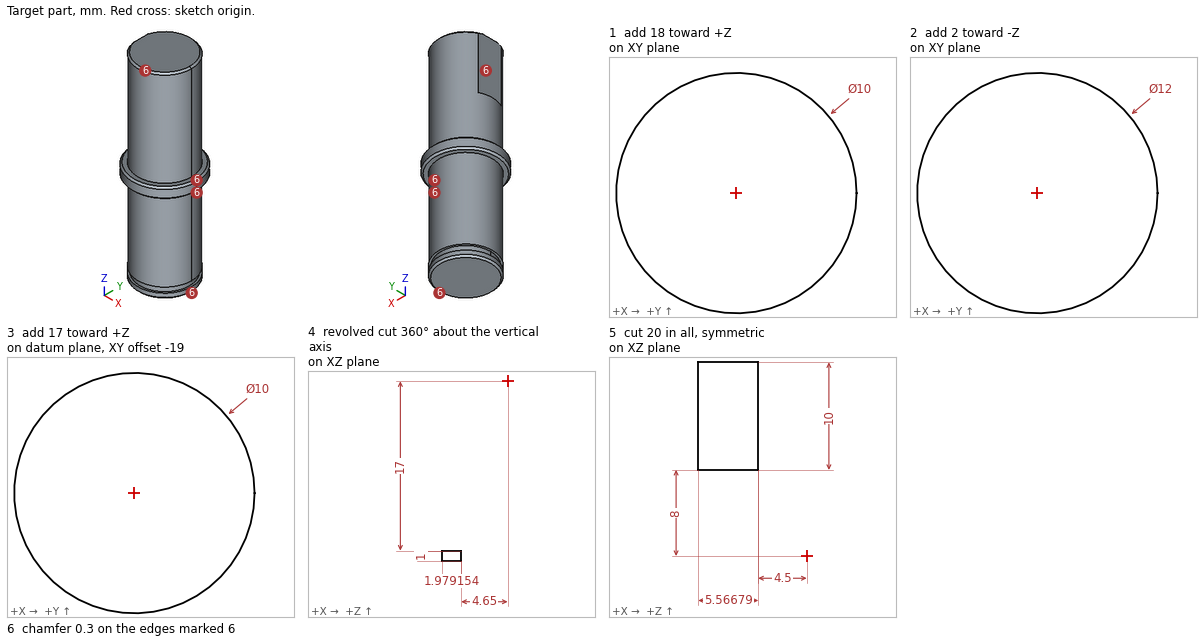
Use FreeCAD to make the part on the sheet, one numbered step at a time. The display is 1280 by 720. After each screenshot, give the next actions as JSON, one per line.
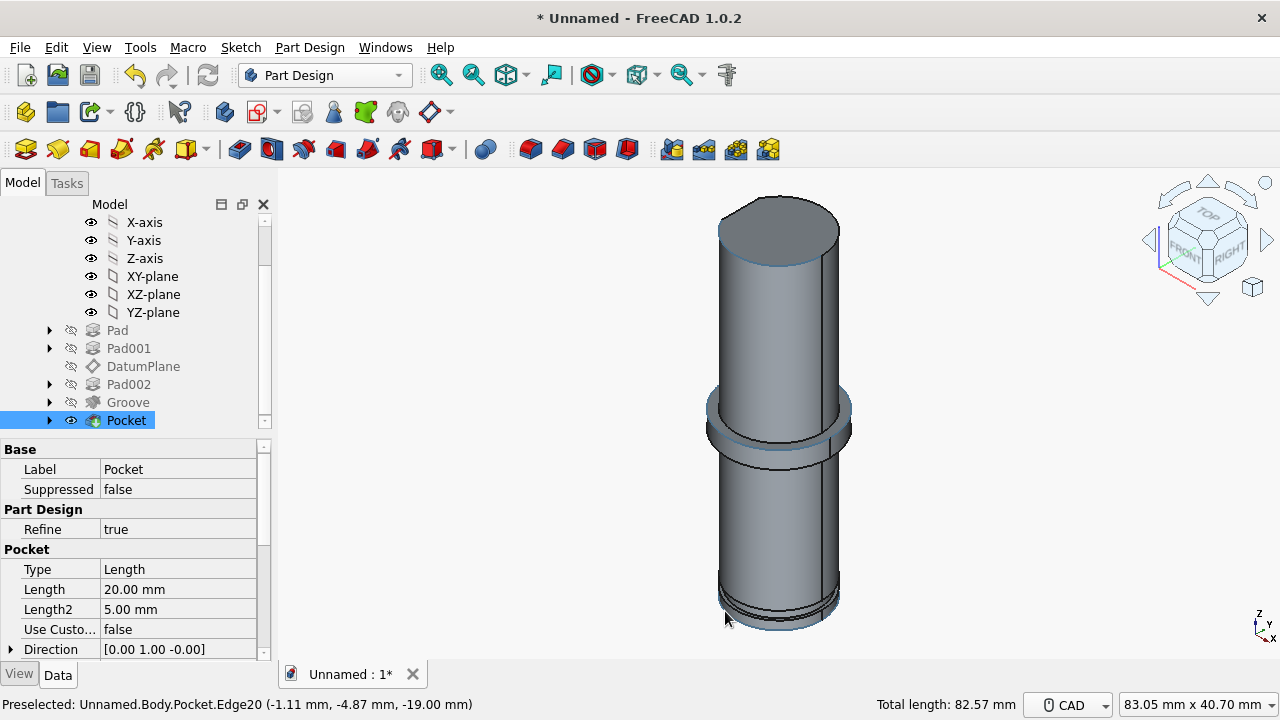
{"action": "key", "text": "2"}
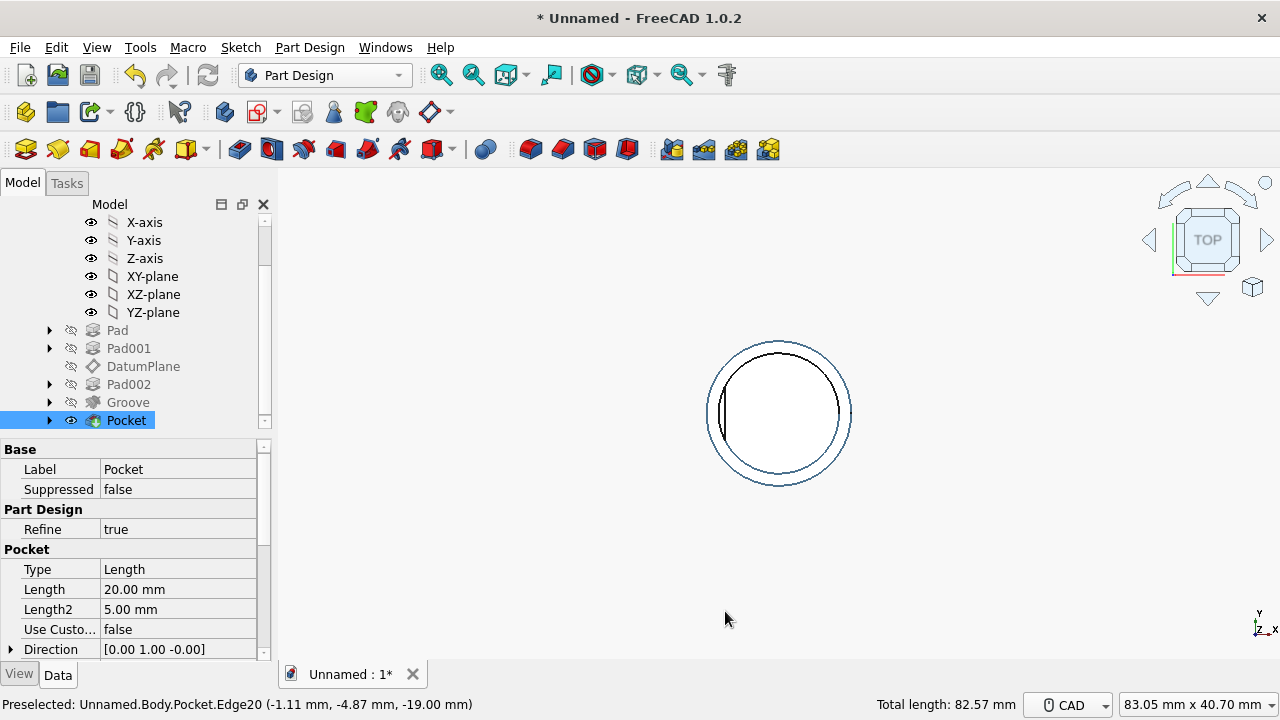
{"action": "left_click", "coordinate": [442, 76]}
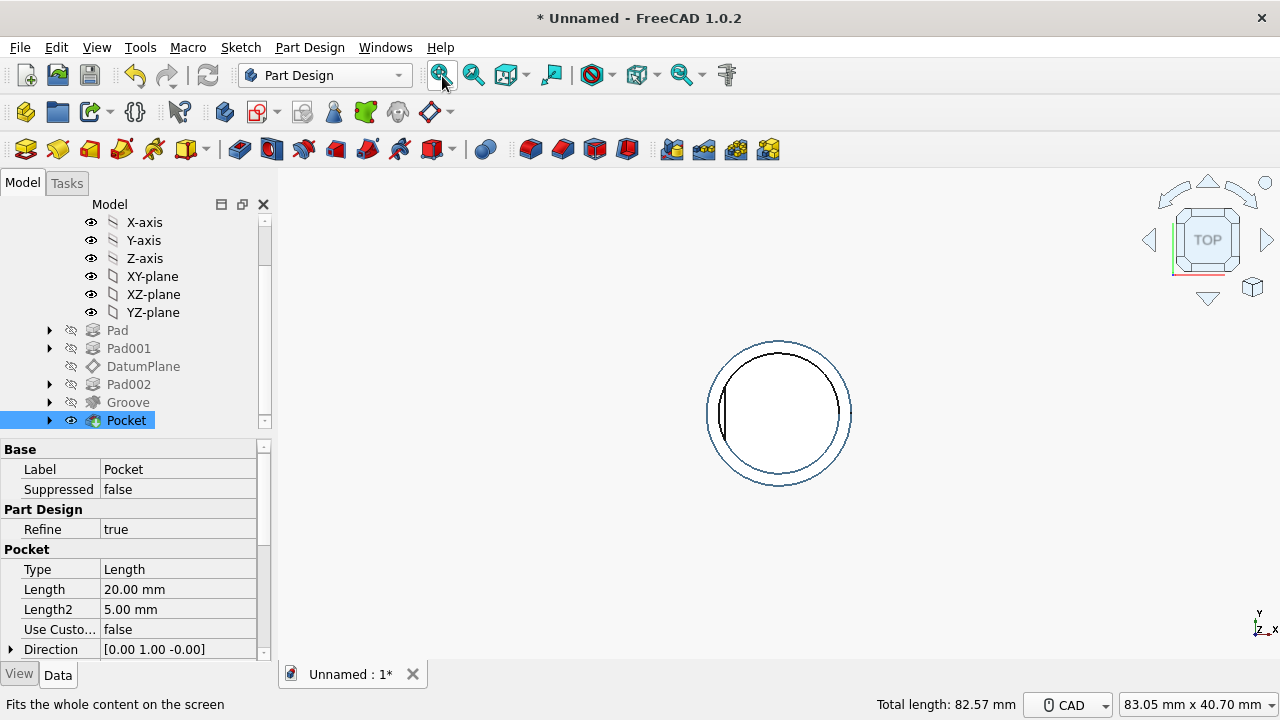
{"action": "key", "text": "1"}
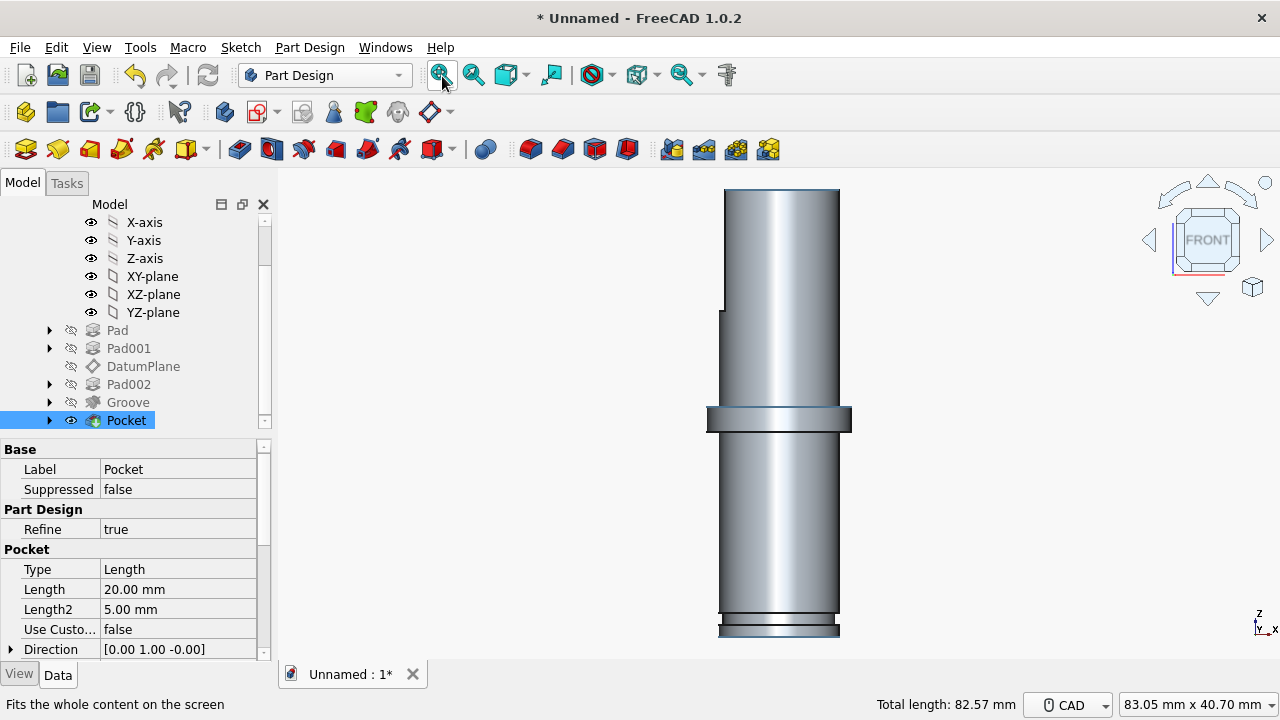
{"action": "left_click", "coordinate": [720, 431], "text": "ctrl"}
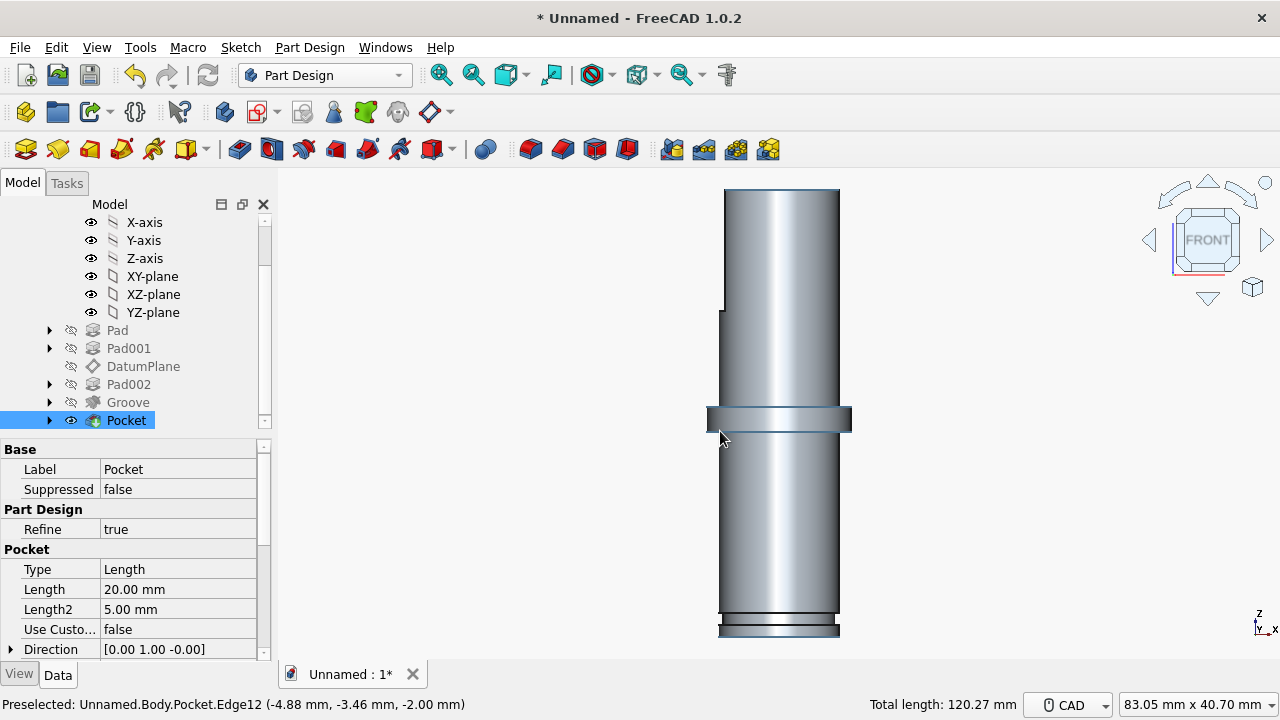
{"action": "left_click", "coordinate": [564, 150]}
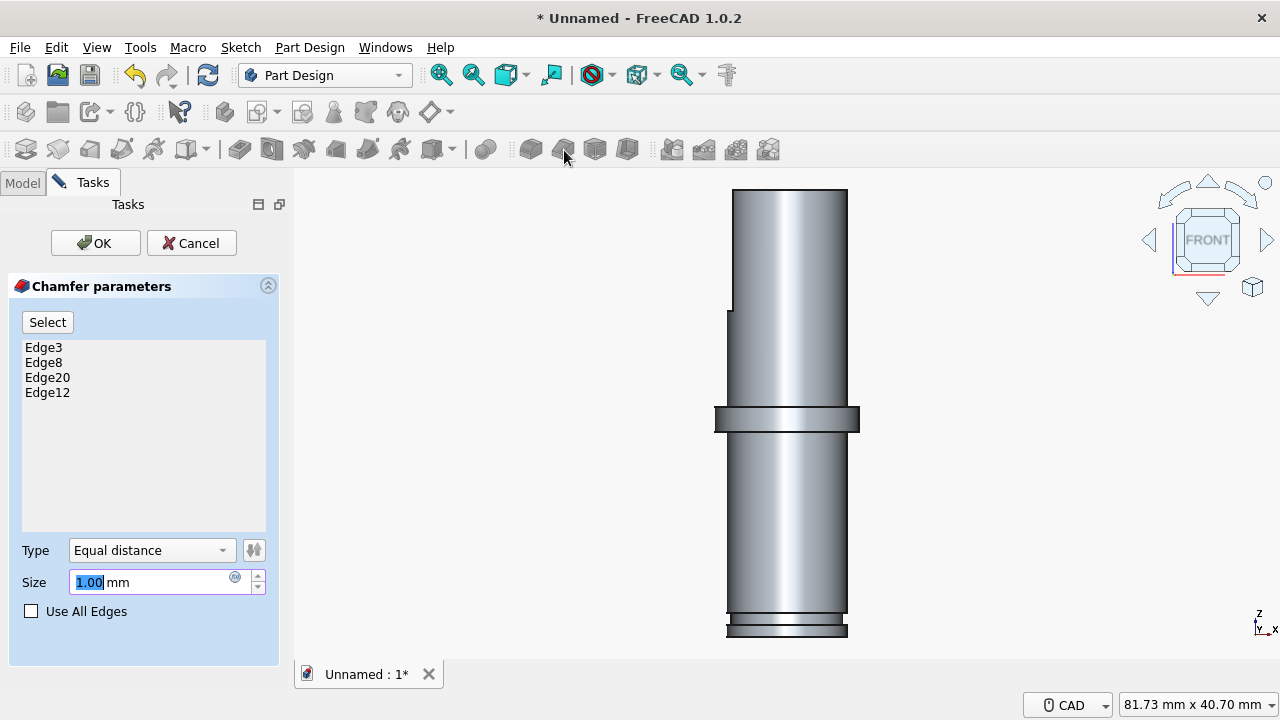
{"action": "type", "text": "0.3"}
{"action": "key", "text": "Tab"}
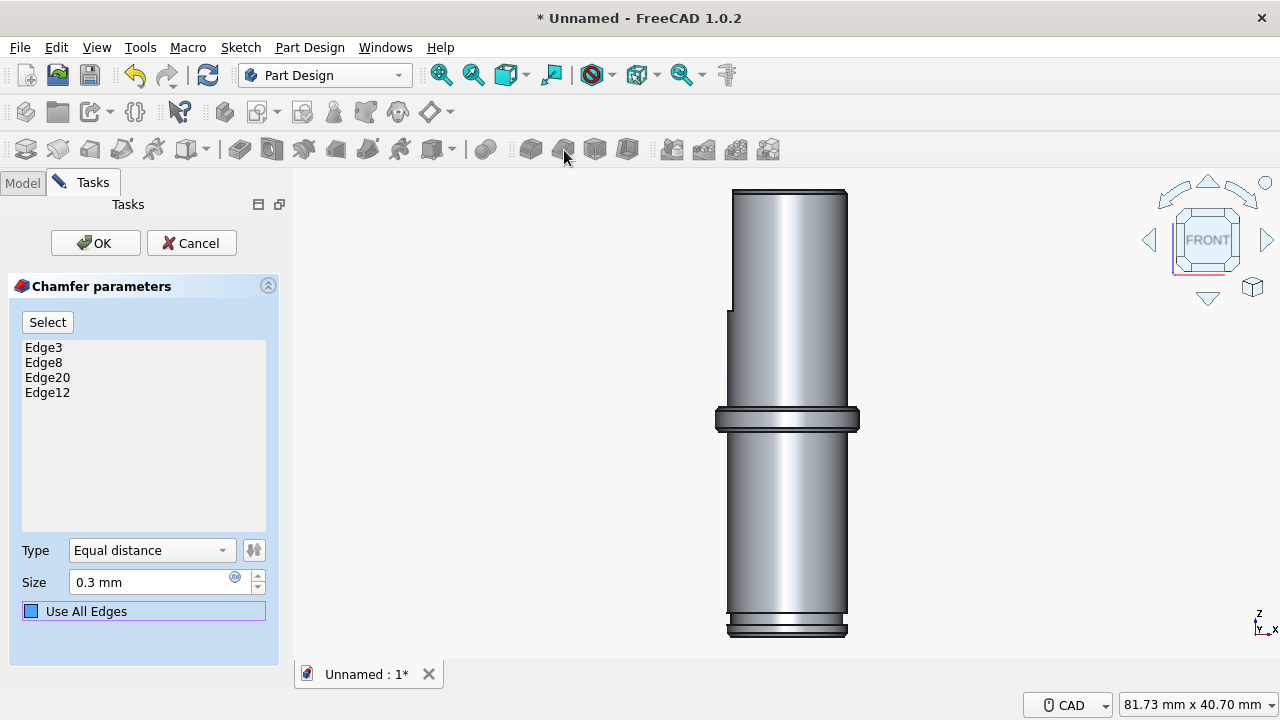
{"action": "left_click", "coordinate": [96, 243]}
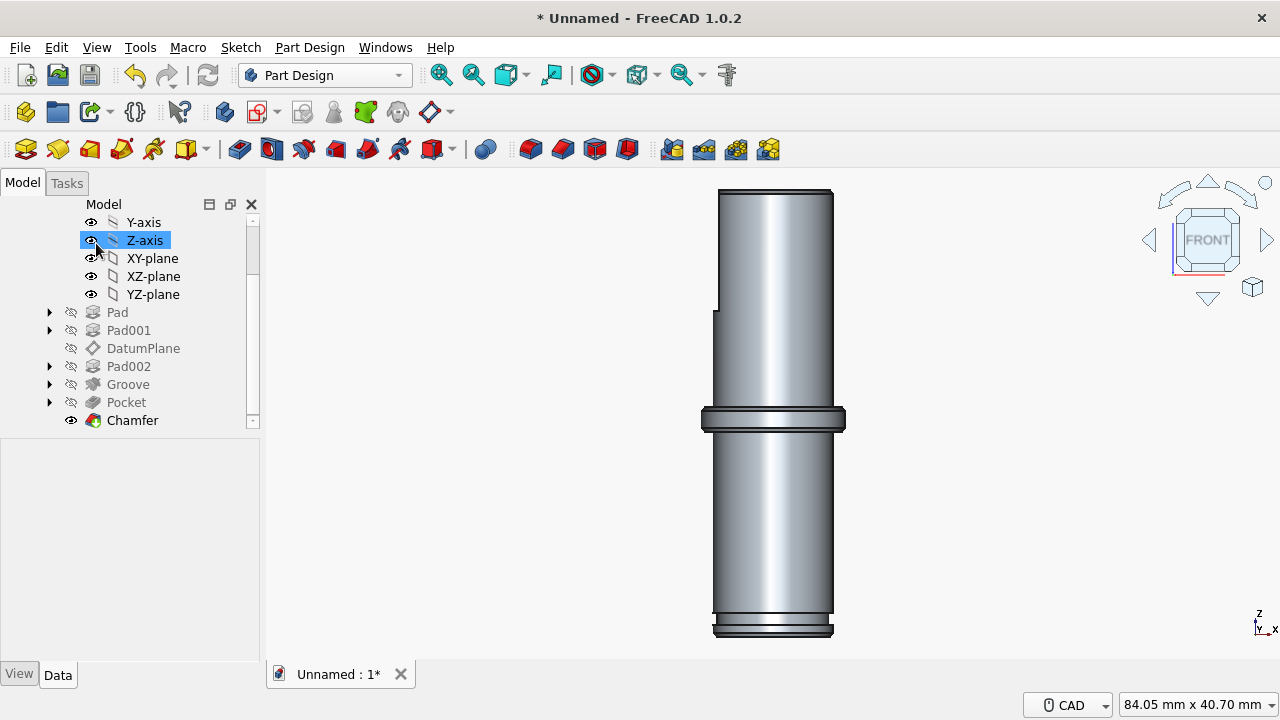
{"action": "key", "text": "0"}